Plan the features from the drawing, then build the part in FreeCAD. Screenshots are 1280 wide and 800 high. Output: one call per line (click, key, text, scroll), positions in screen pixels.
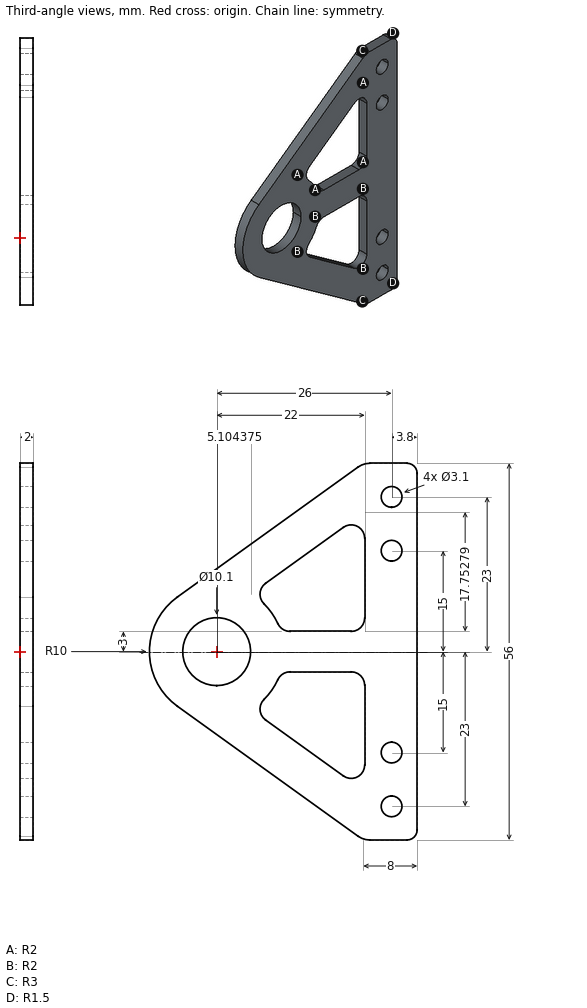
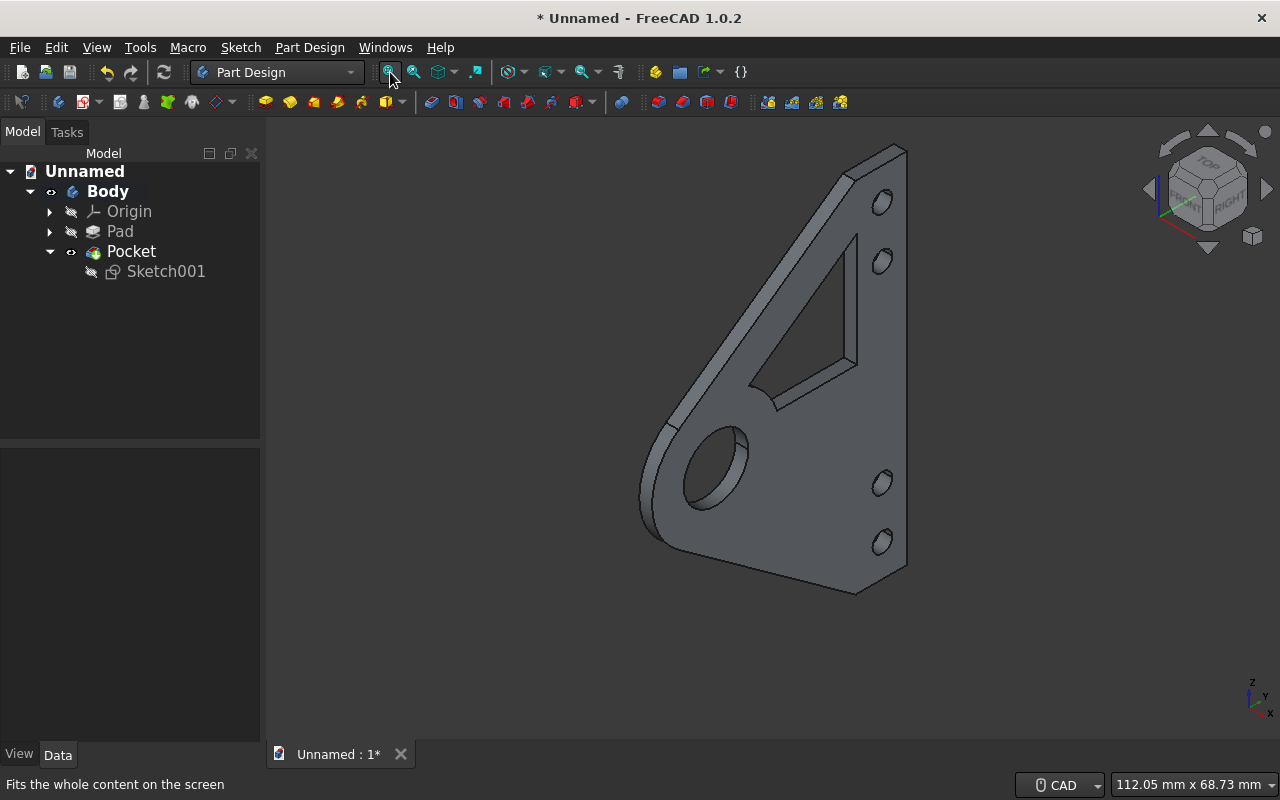
key(2)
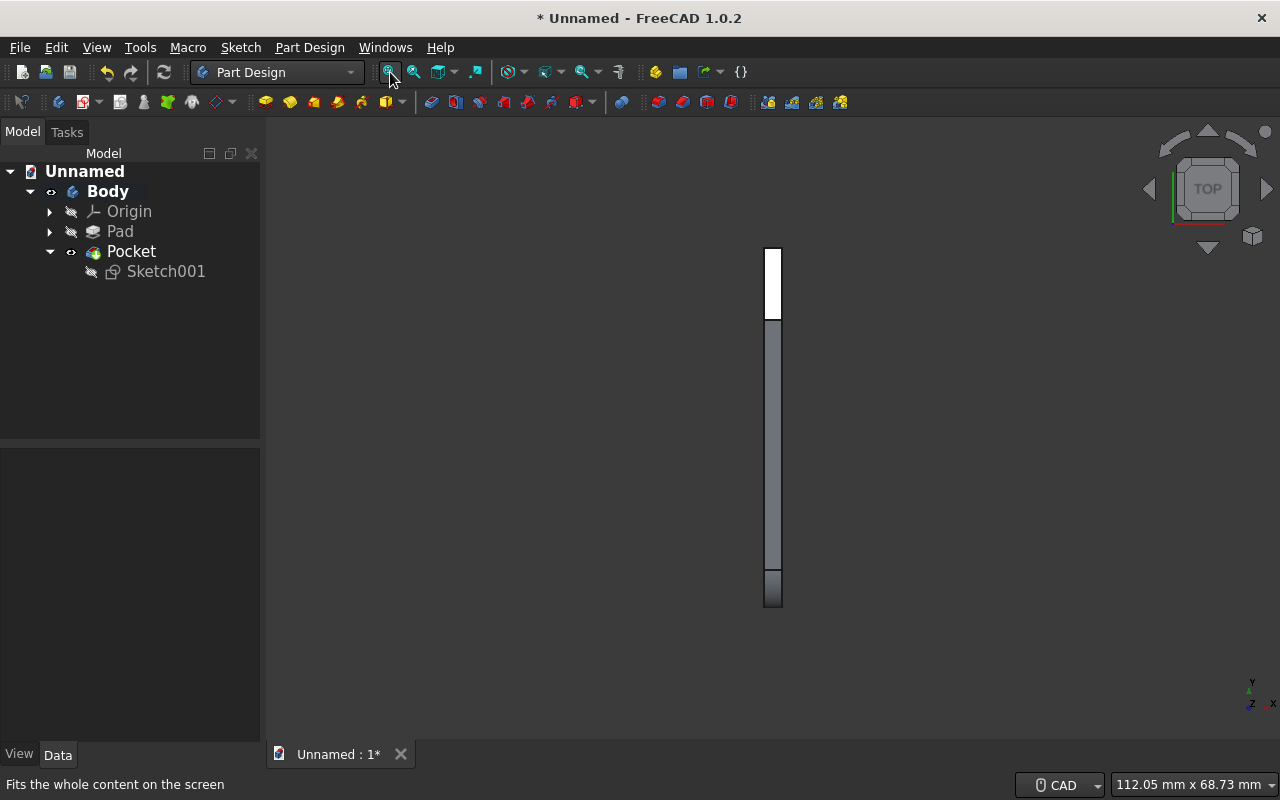
scroll(773, 317, up, 4)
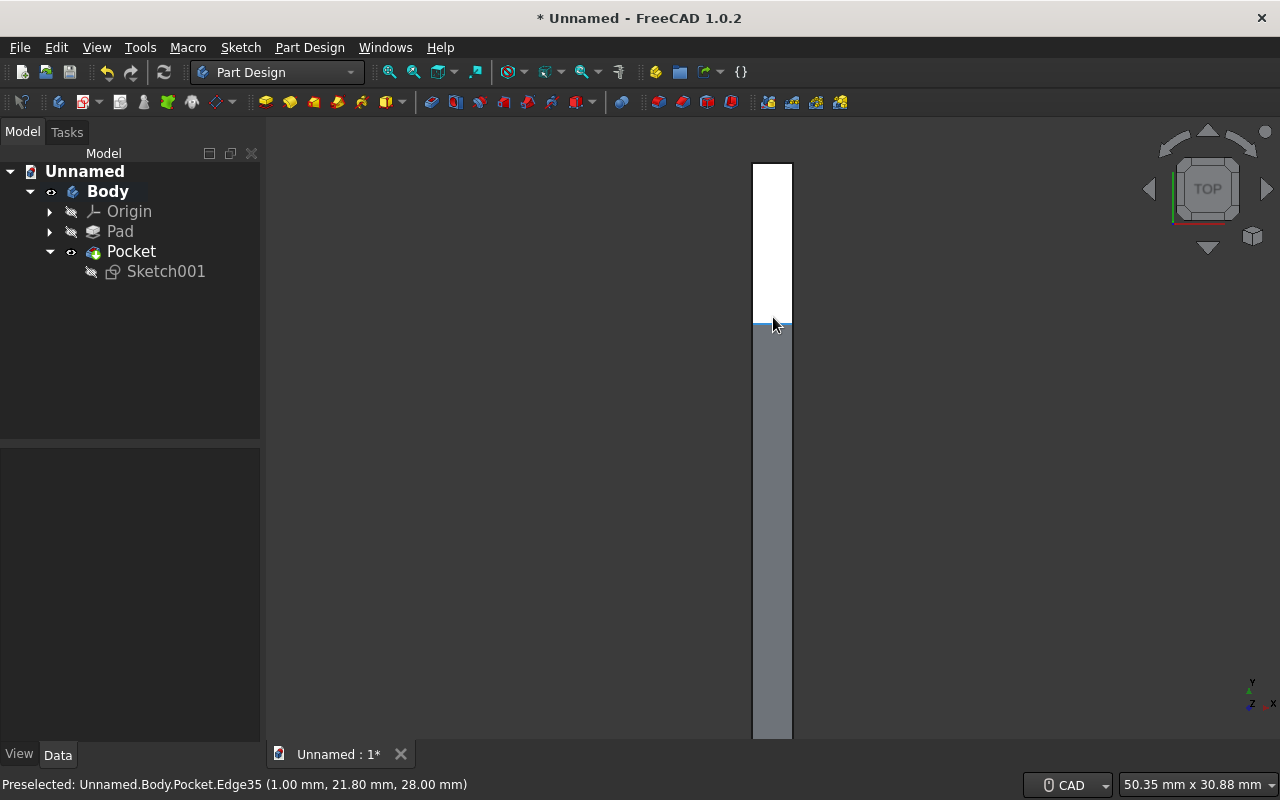
click(390, 72)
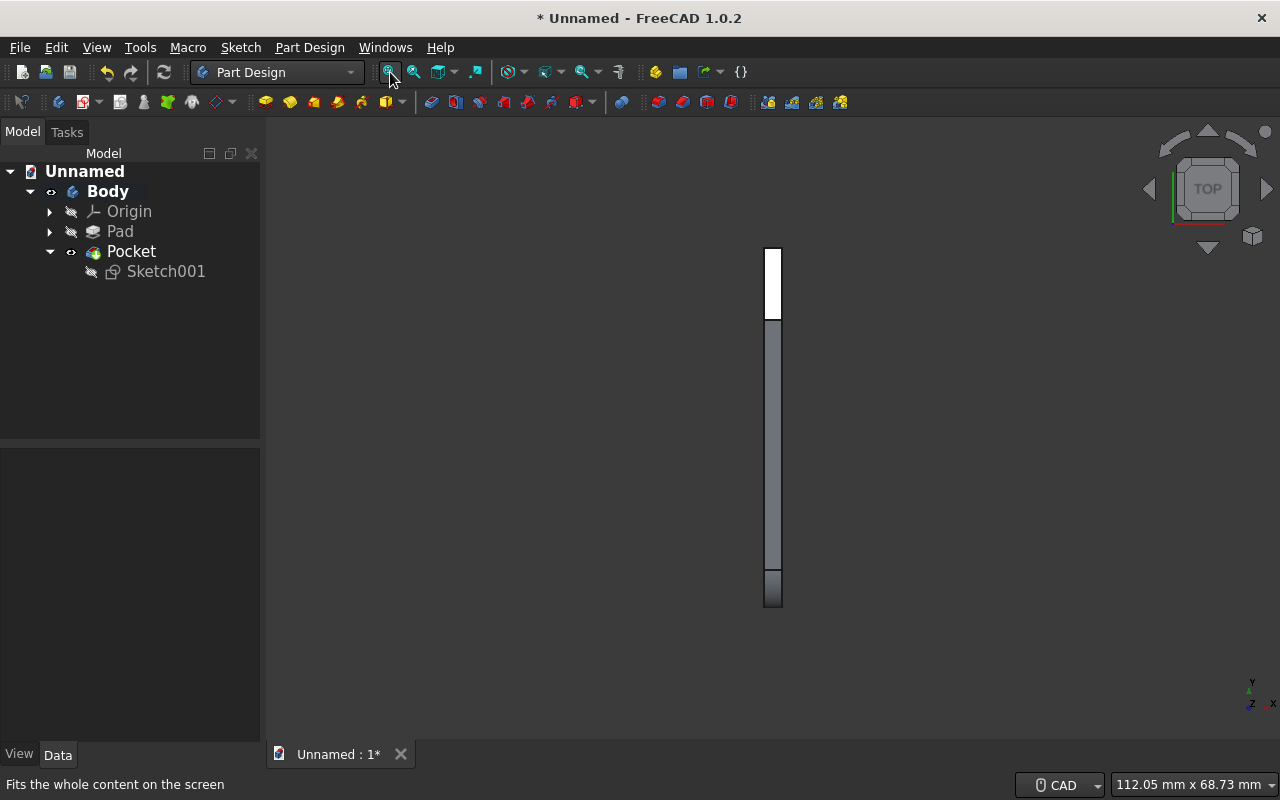
key(1)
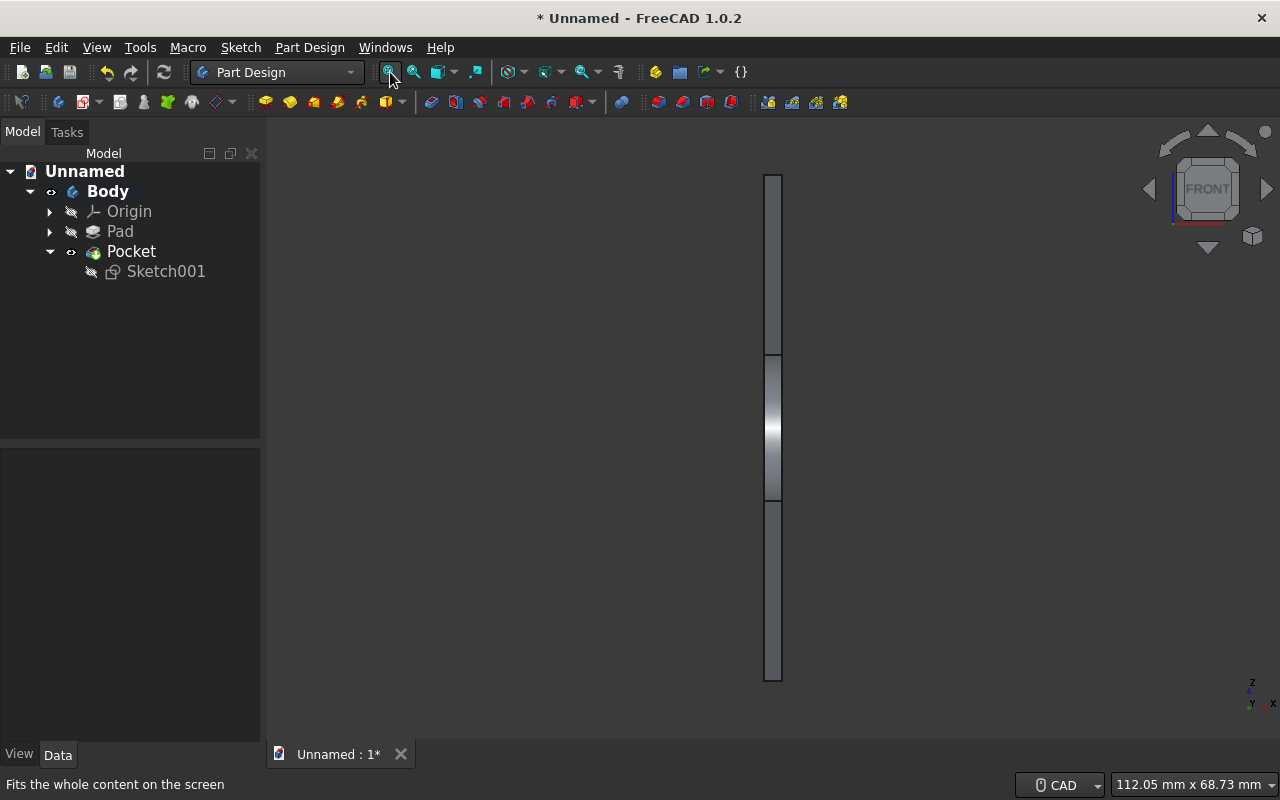
scroll(773, 400, up, 4)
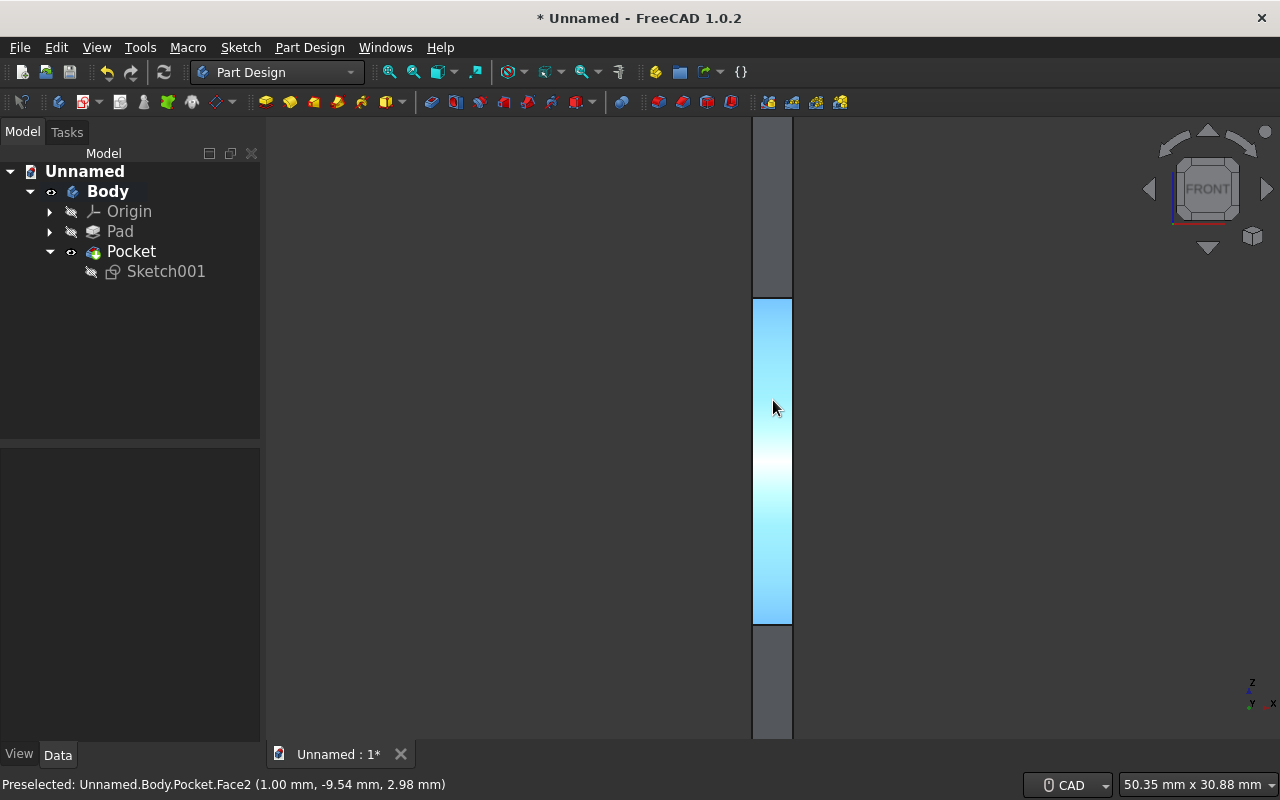
click(390, 72)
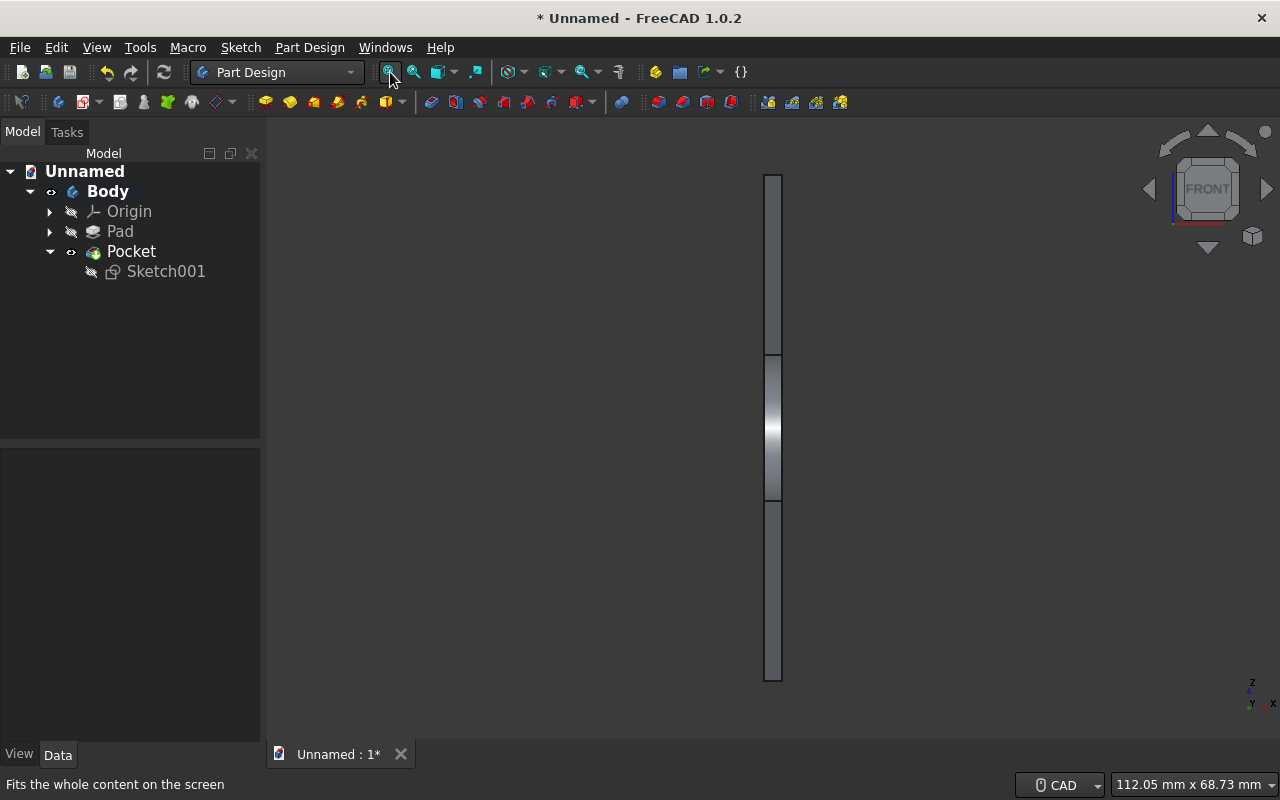
key(3)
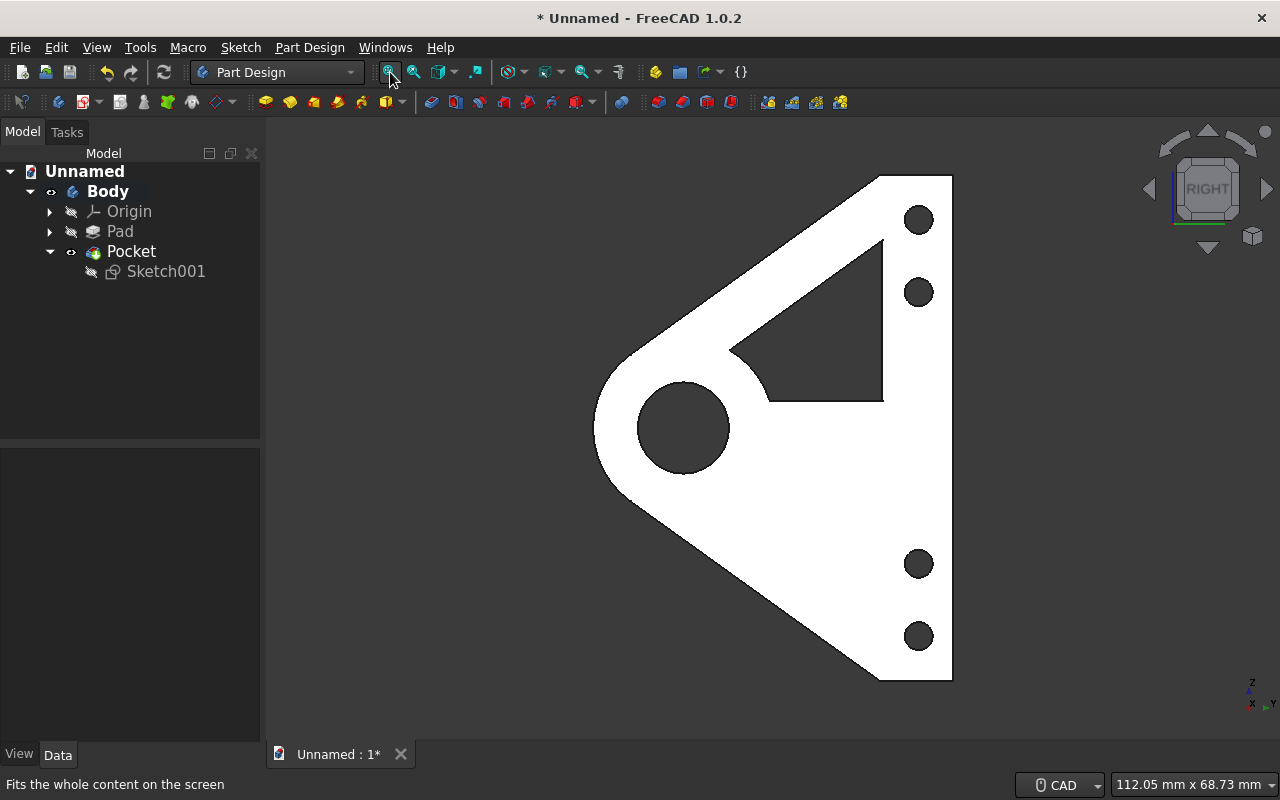
scroll(883, 400, up, 4)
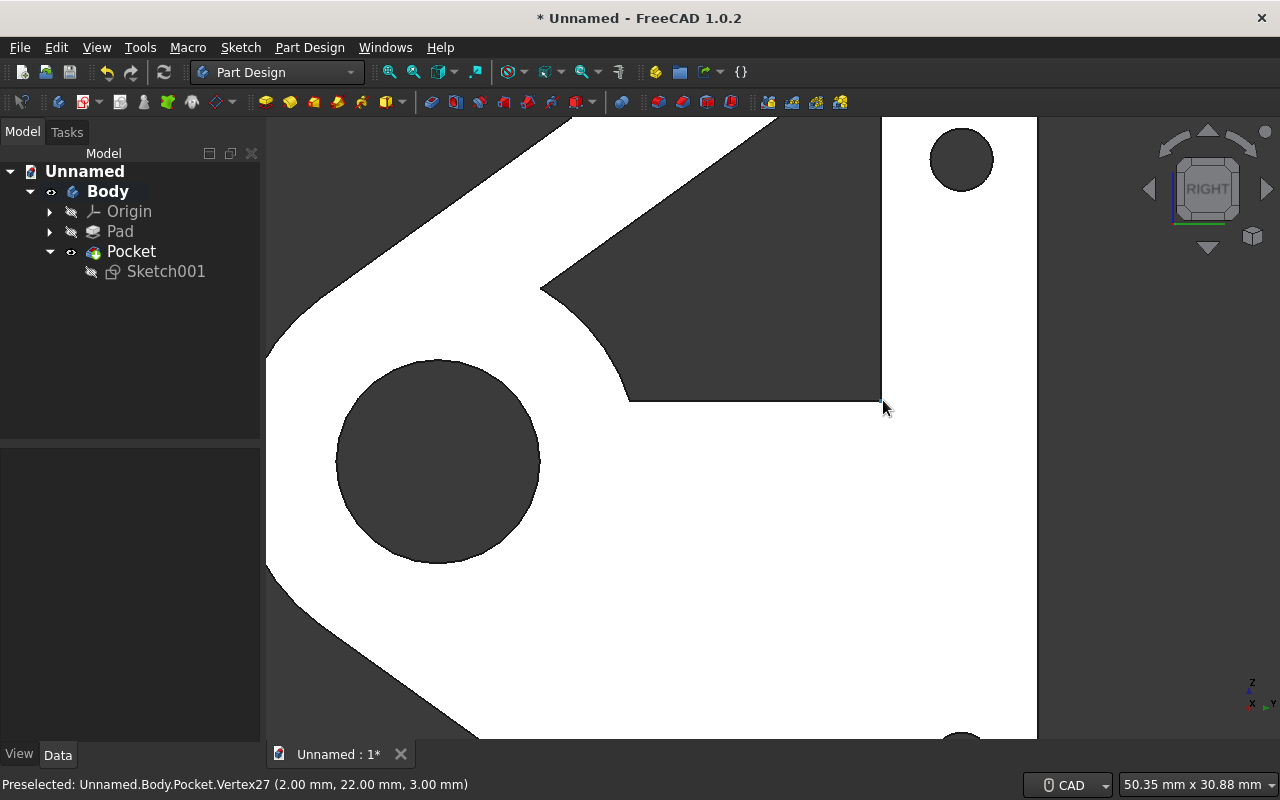
click(390, 72)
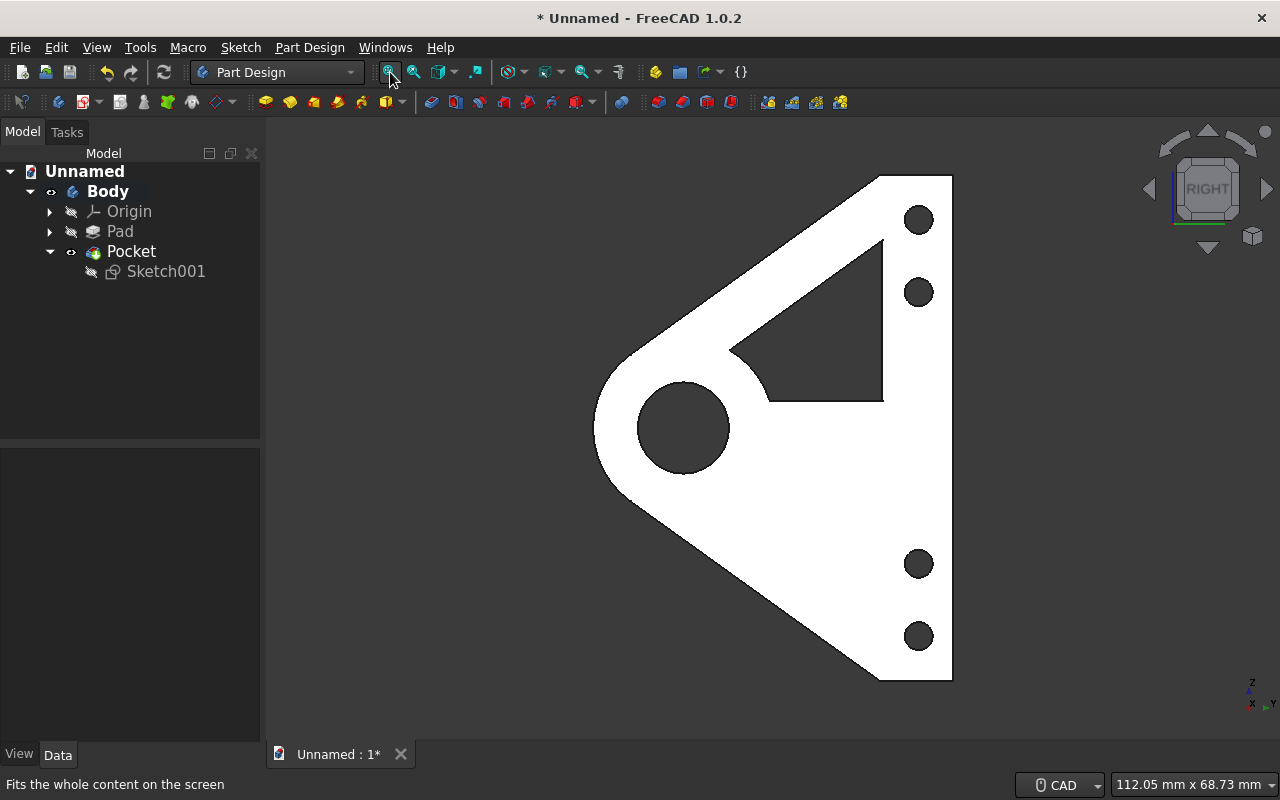
key(5)